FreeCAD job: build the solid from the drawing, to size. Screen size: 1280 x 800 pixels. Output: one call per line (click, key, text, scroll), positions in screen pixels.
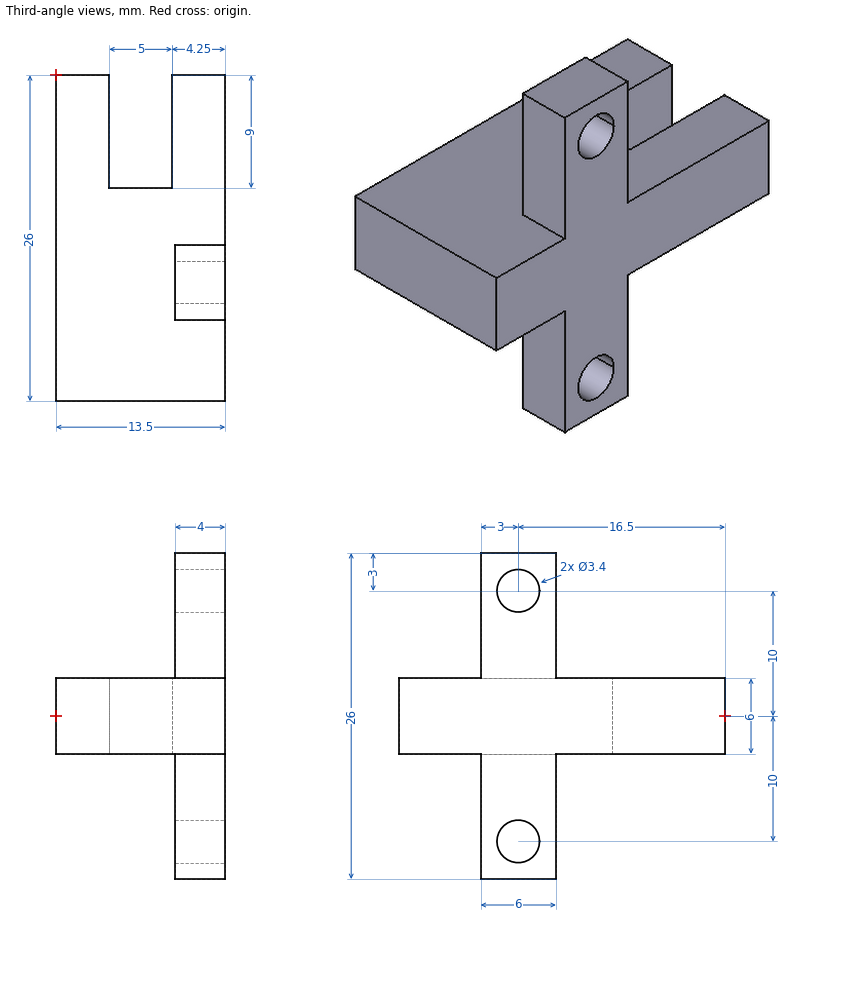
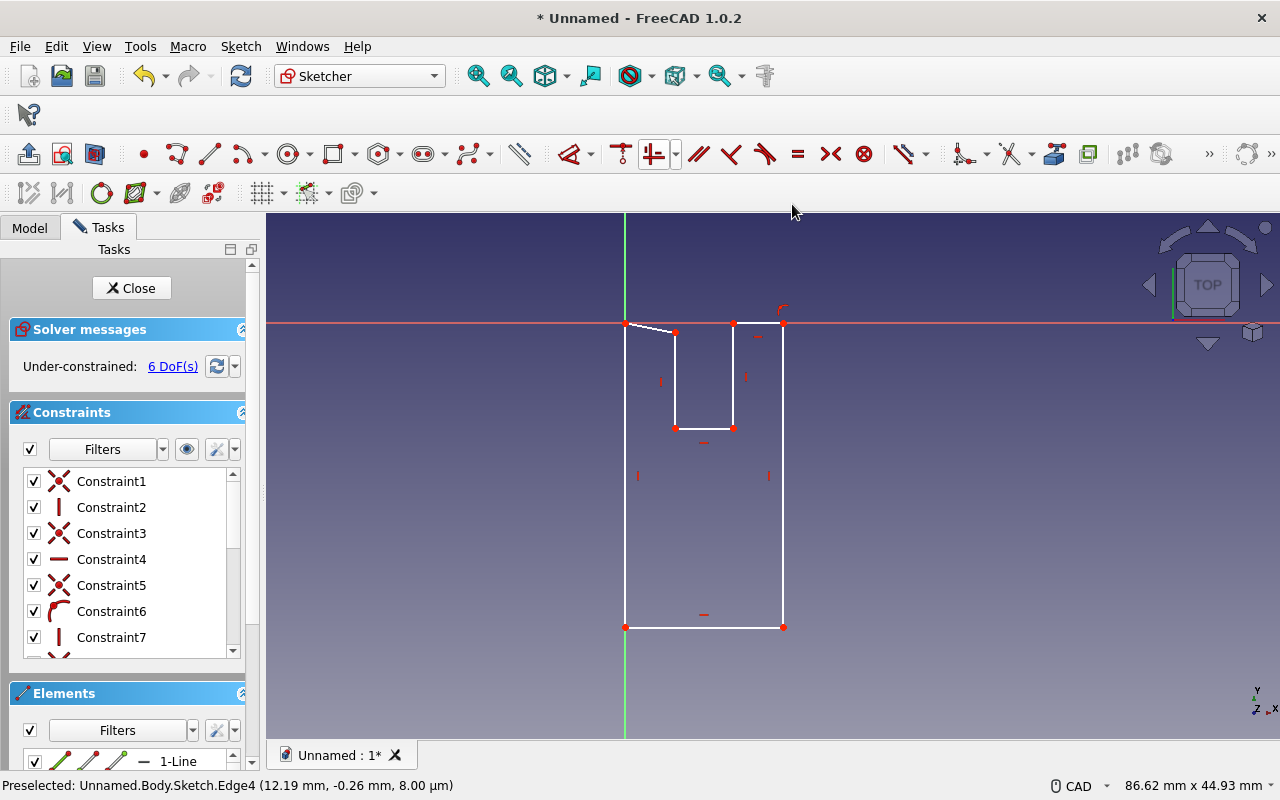
click(640, 326)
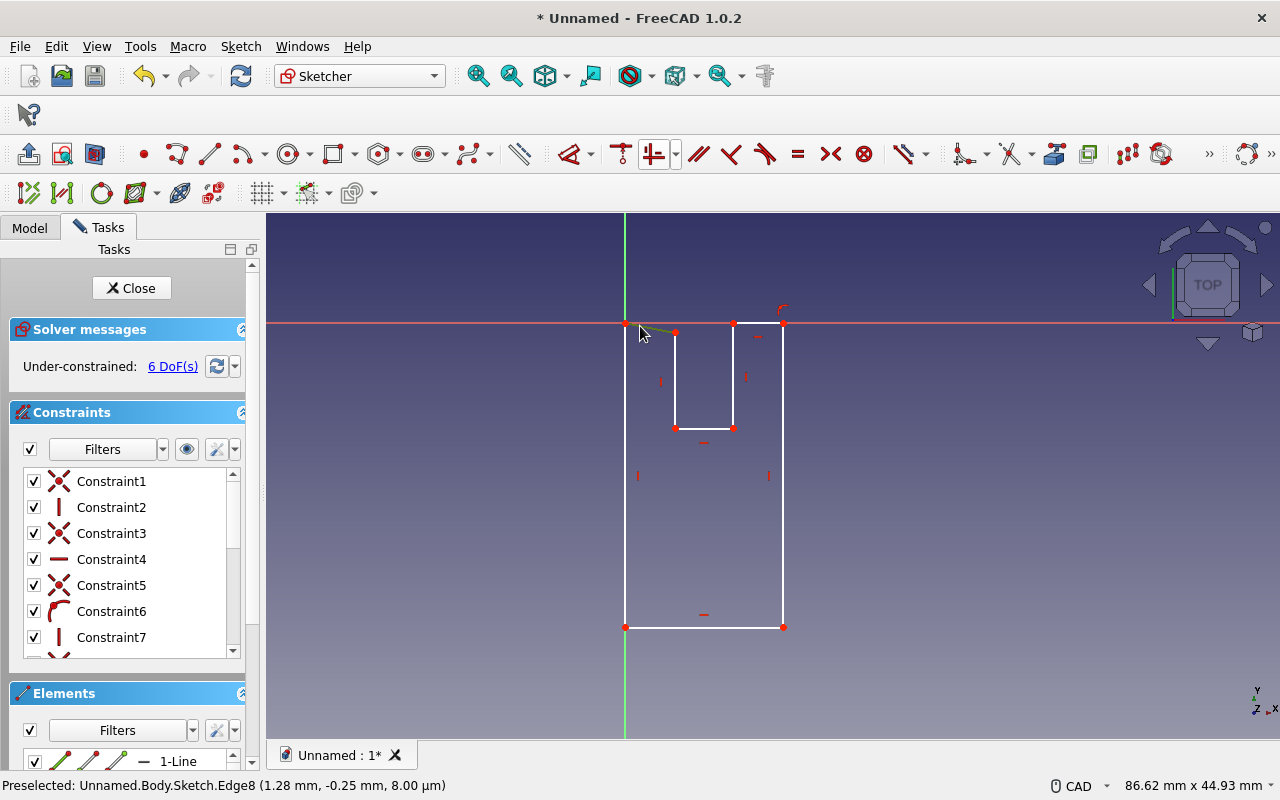
click(676, 154)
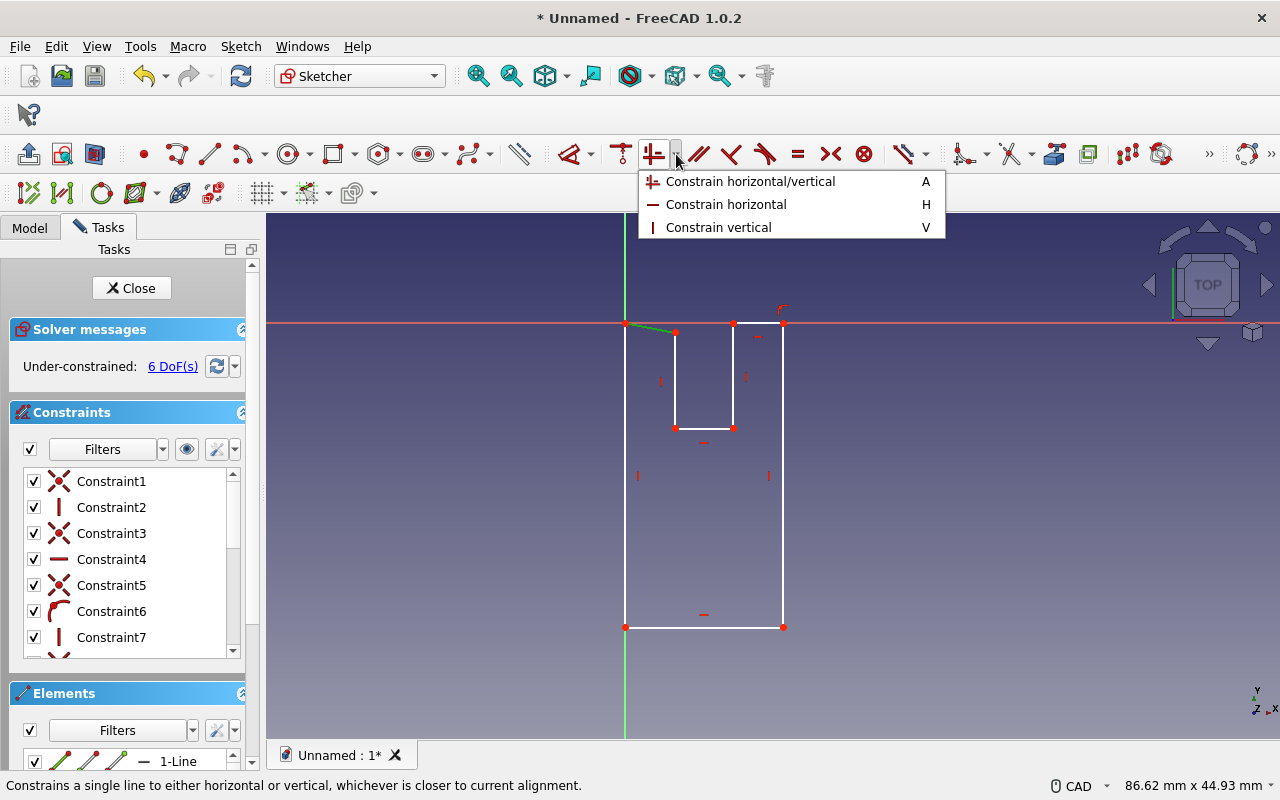
click(792, 204)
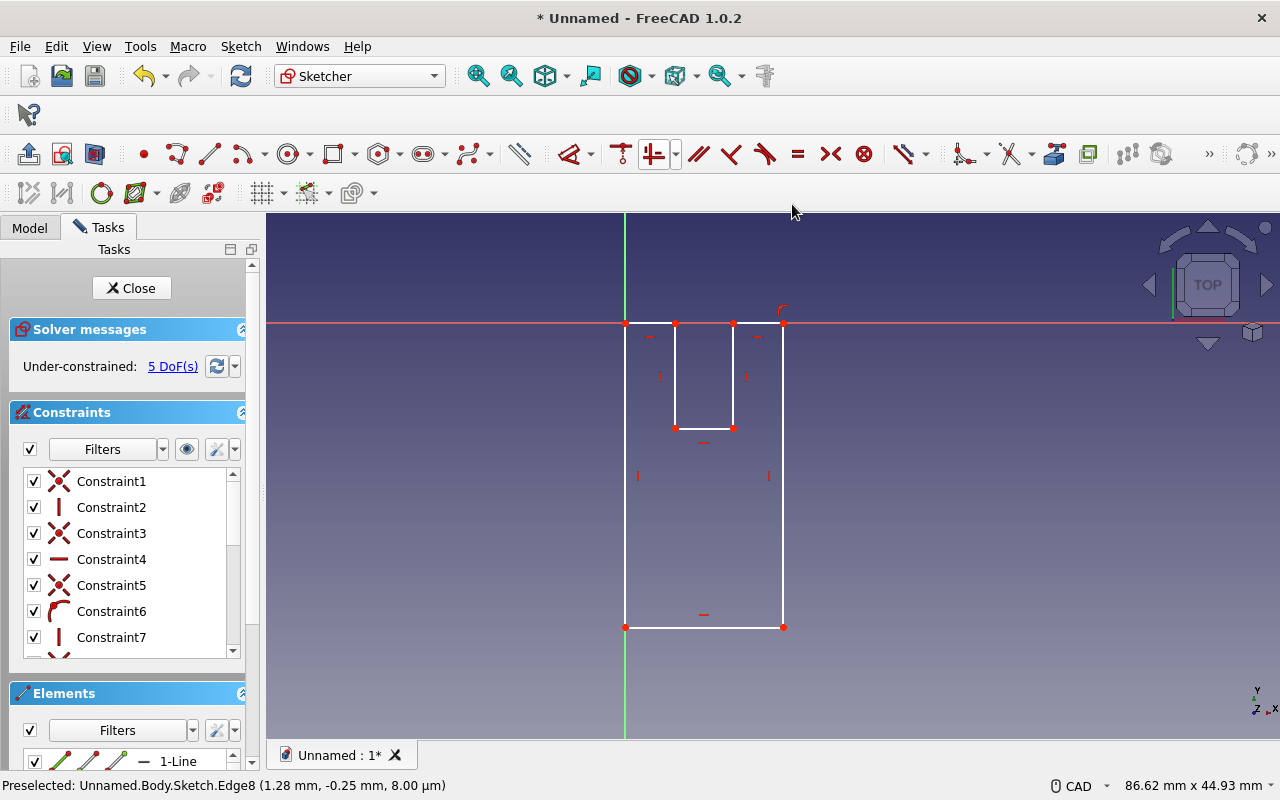
click(568, 154)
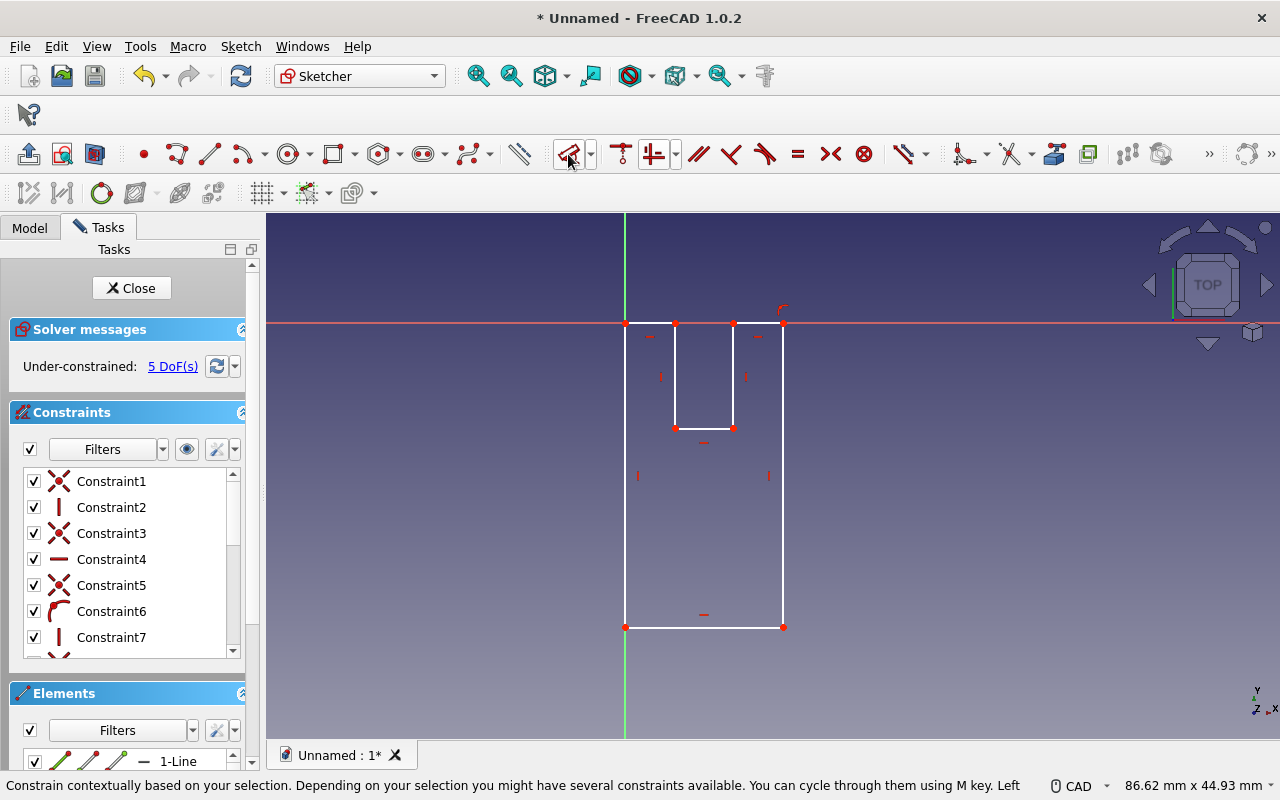
click(733, 355)
click(767, 376)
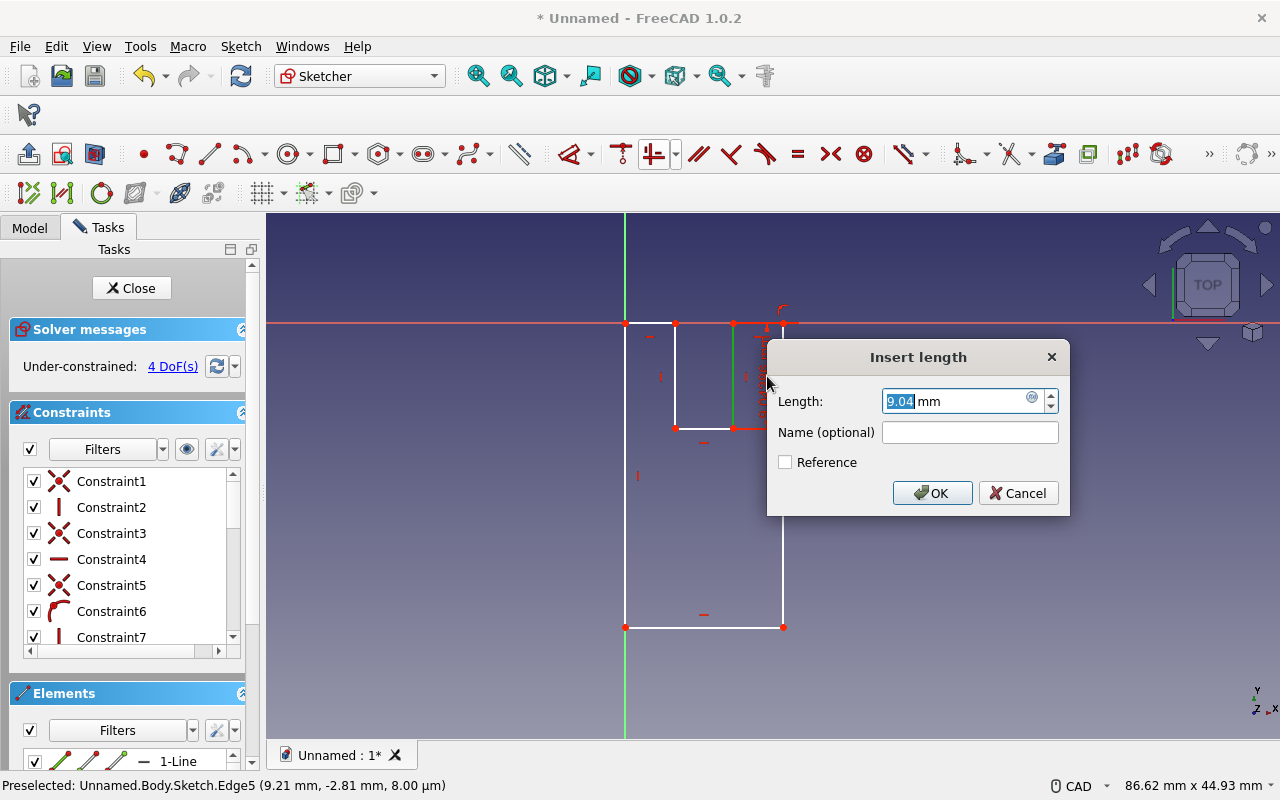
text(9)
key(Return)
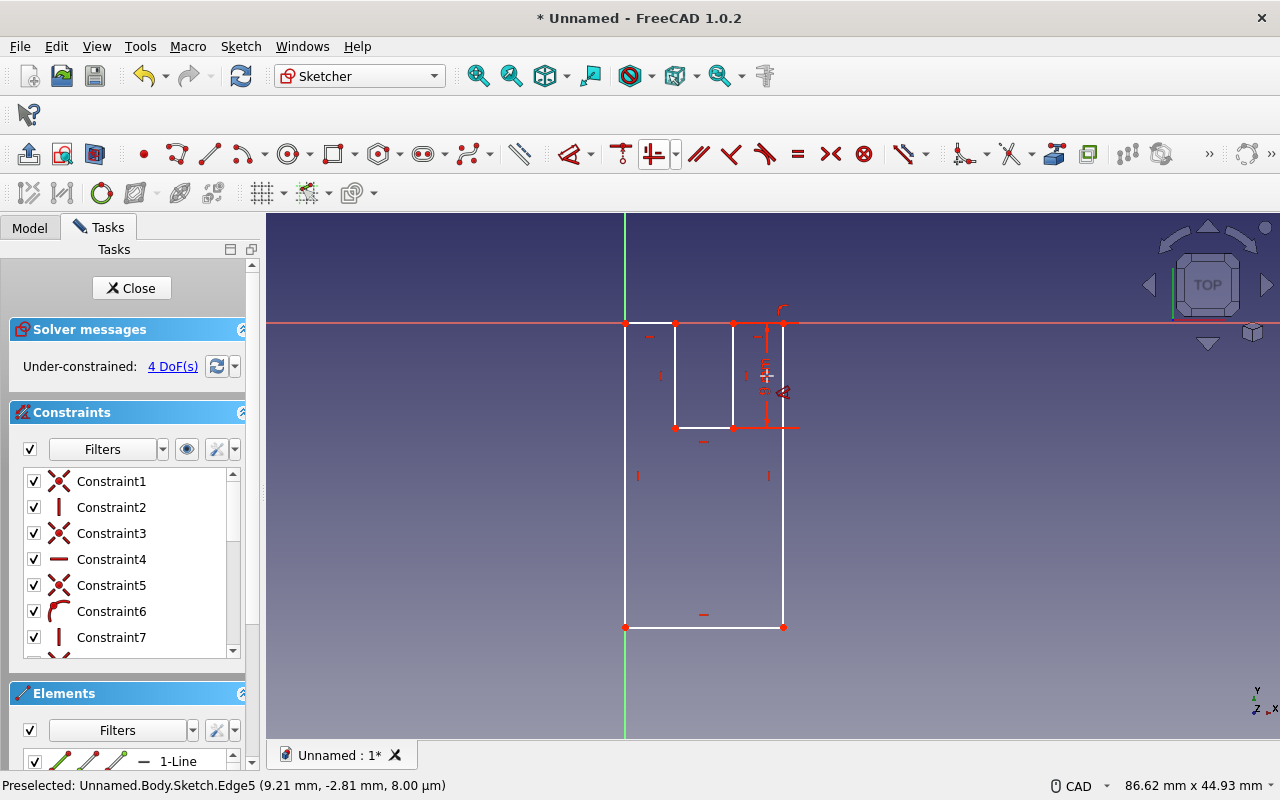
click(716, 428)
click(691, 394)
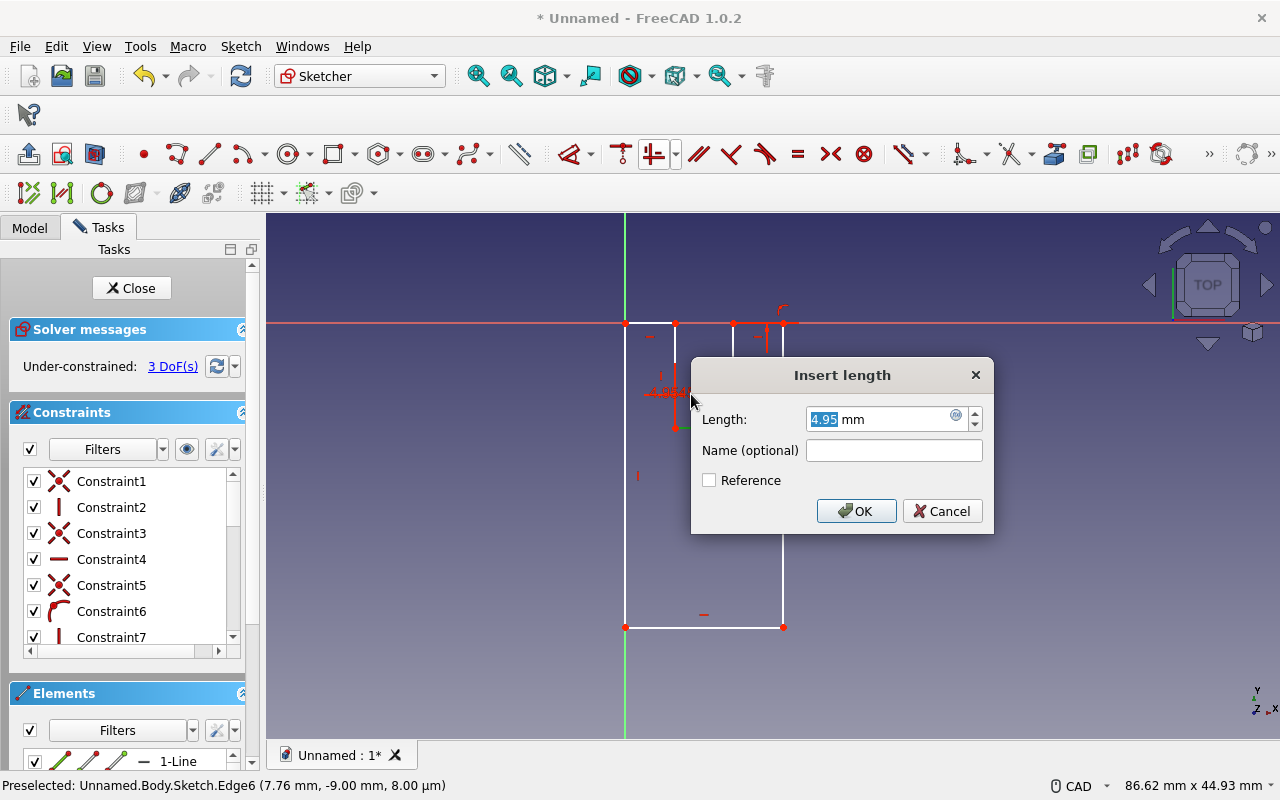
text(5)
key(Return)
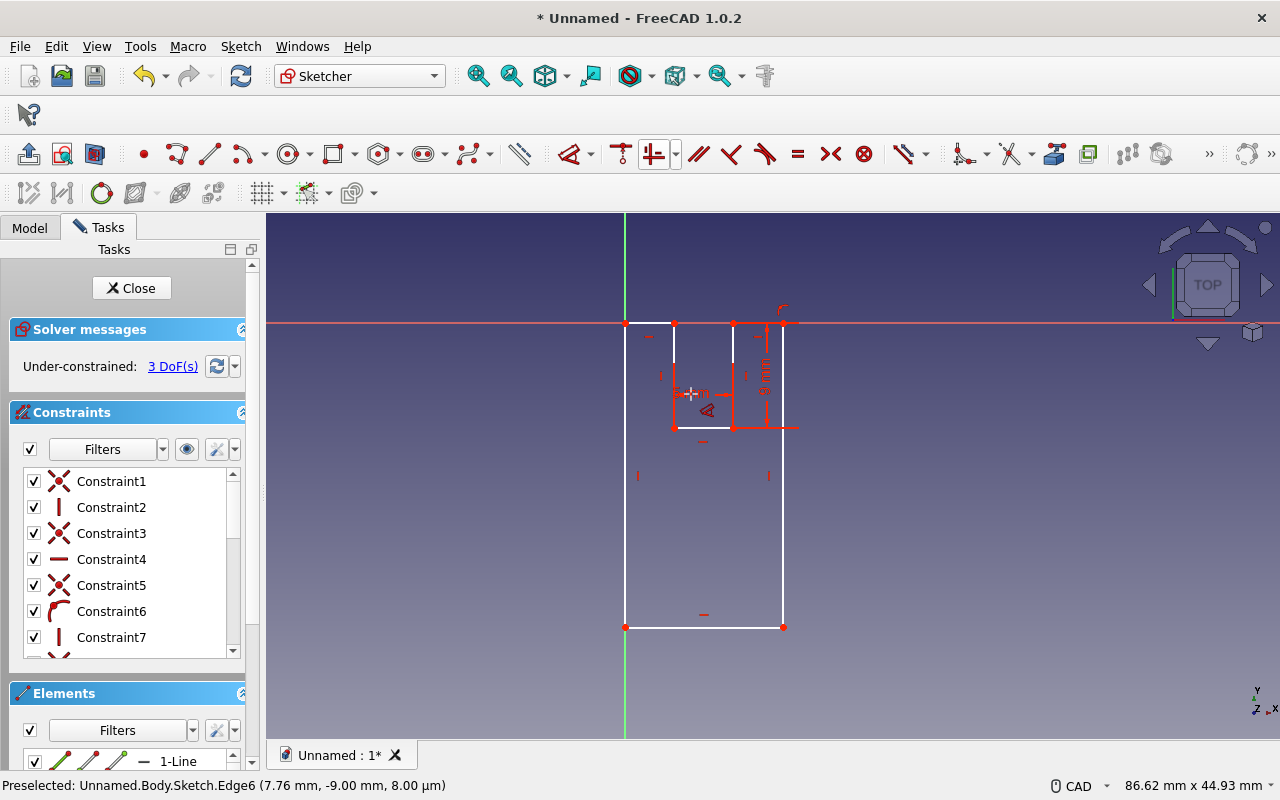
click(625, 415)
click(591, 476)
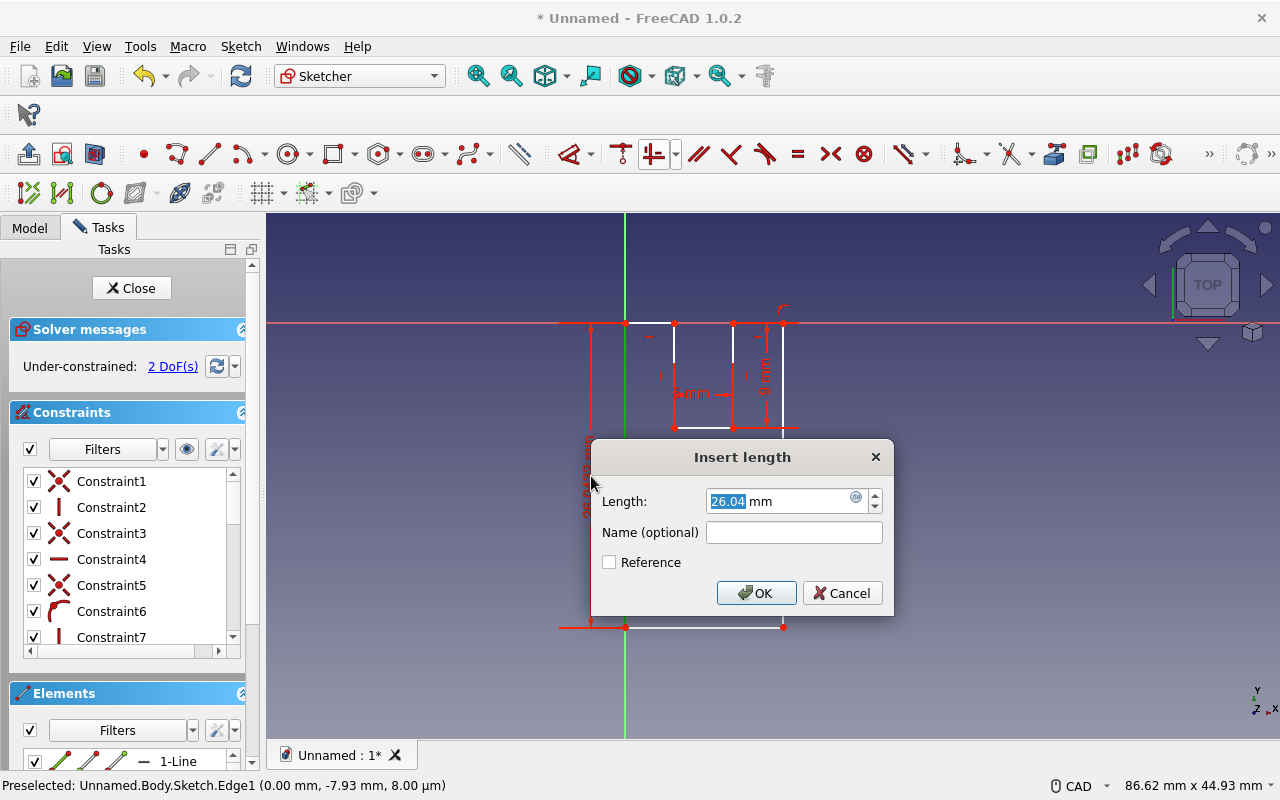
text(26)
key(Return)